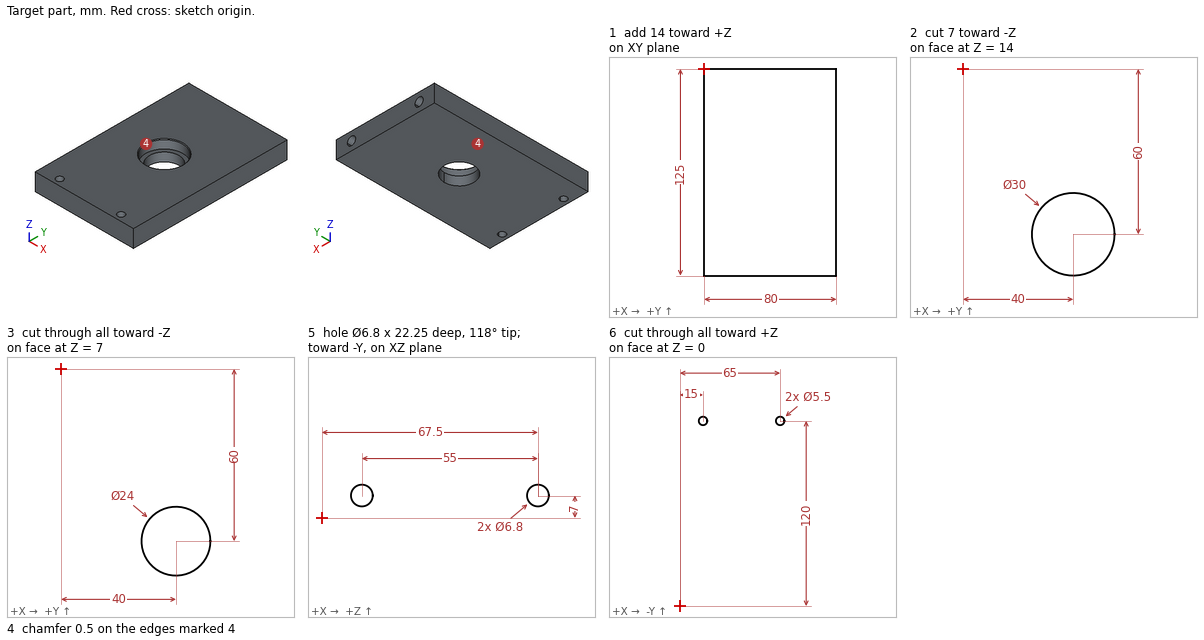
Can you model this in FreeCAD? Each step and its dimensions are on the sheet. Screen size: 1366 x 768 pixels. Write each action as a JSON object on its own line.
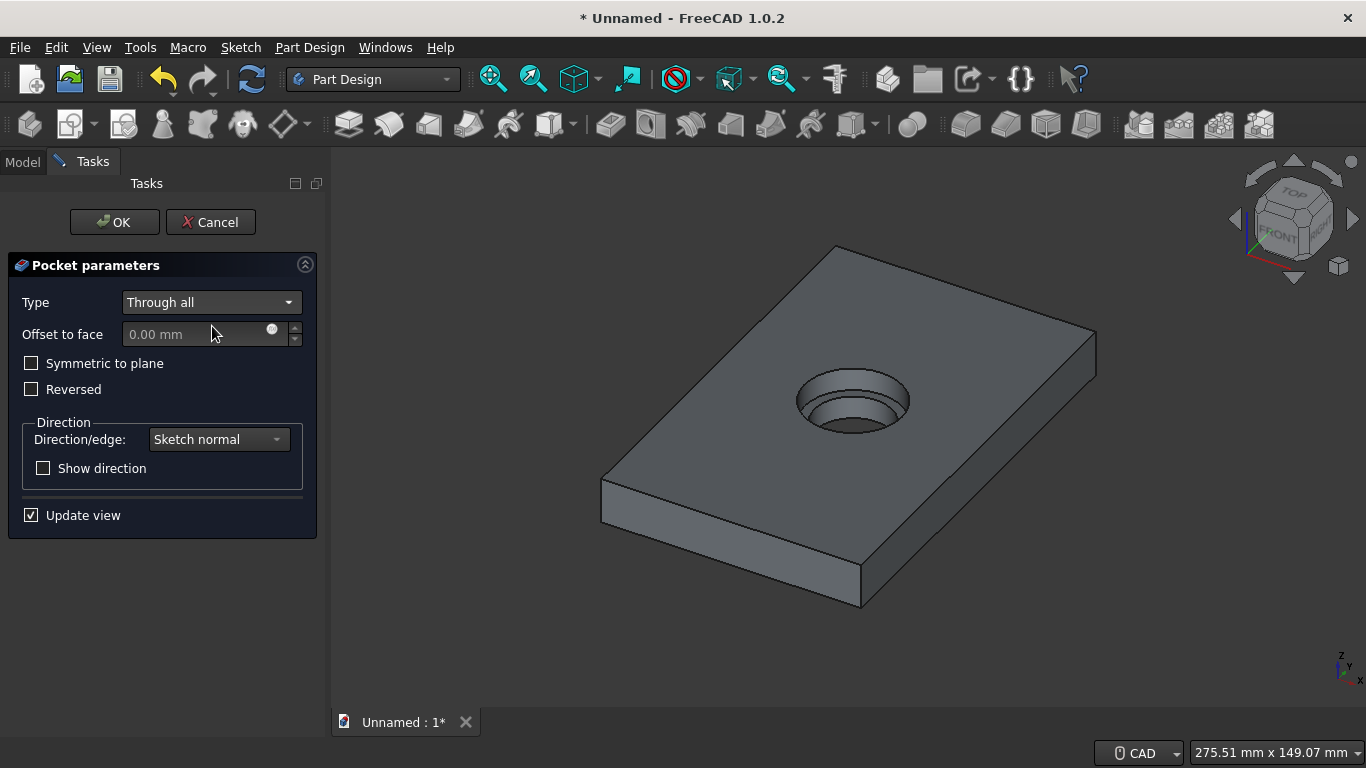
{"action": "left_click", "coordinate": [115, 222]}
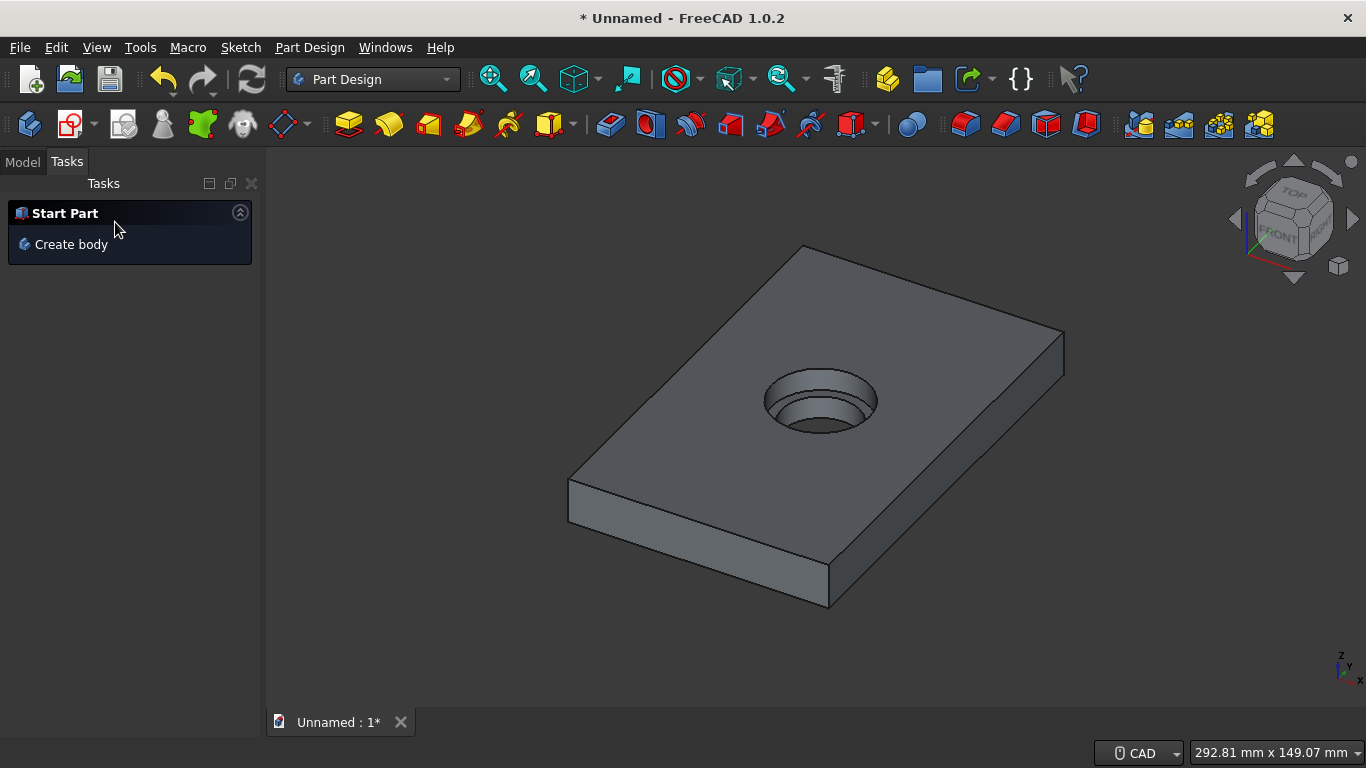
{"action": "left_click", "coordinate": [772, 384]}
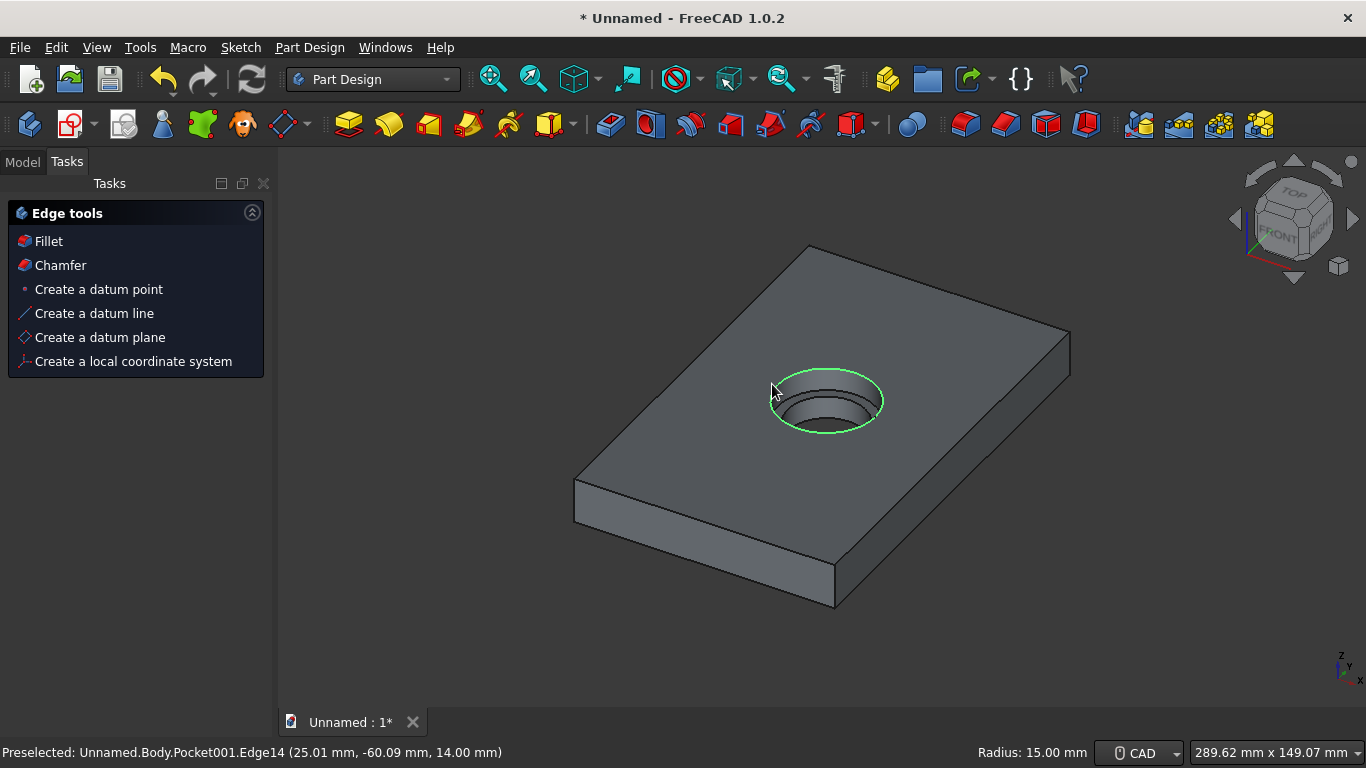
{"action": "left_click", "coordinate": [1006, 124]}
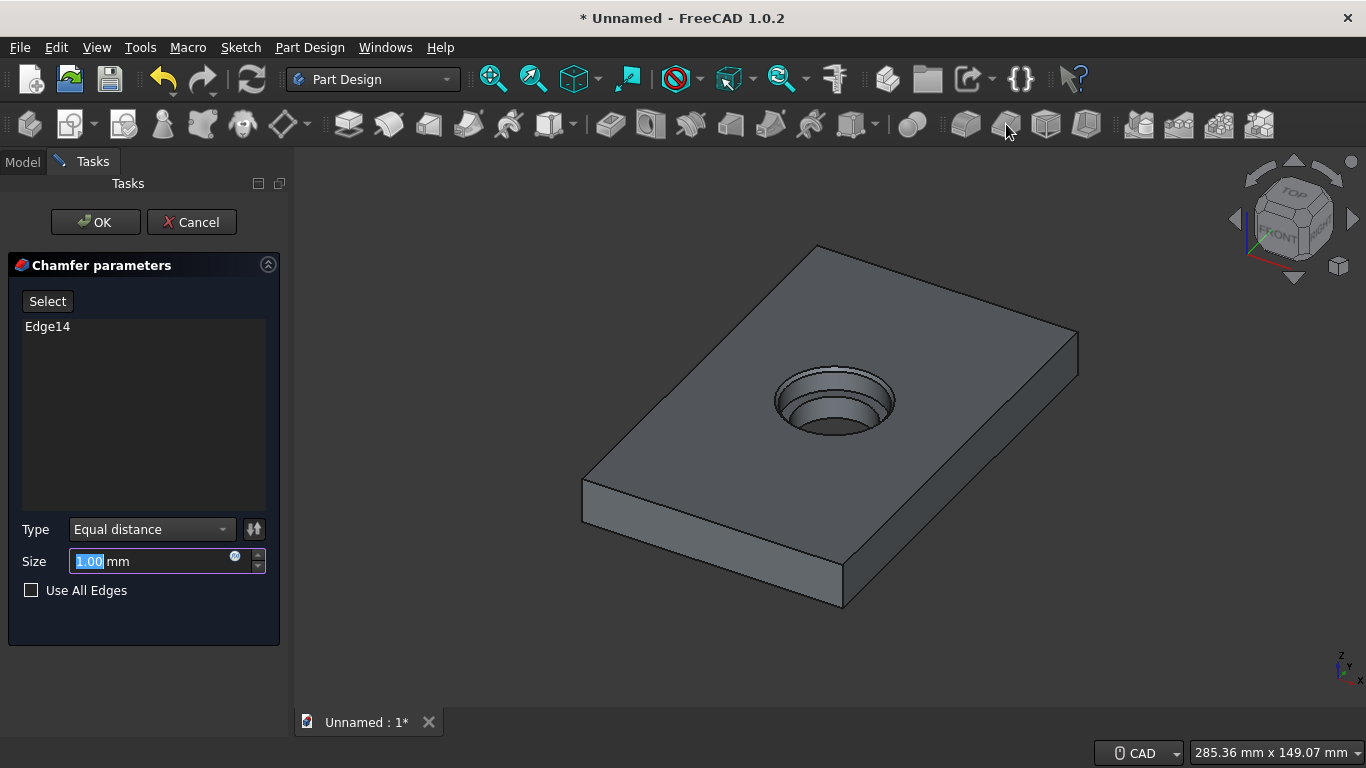
{"action": "type", "text": "0.5"}
{"action": "key", "text": "Tab"}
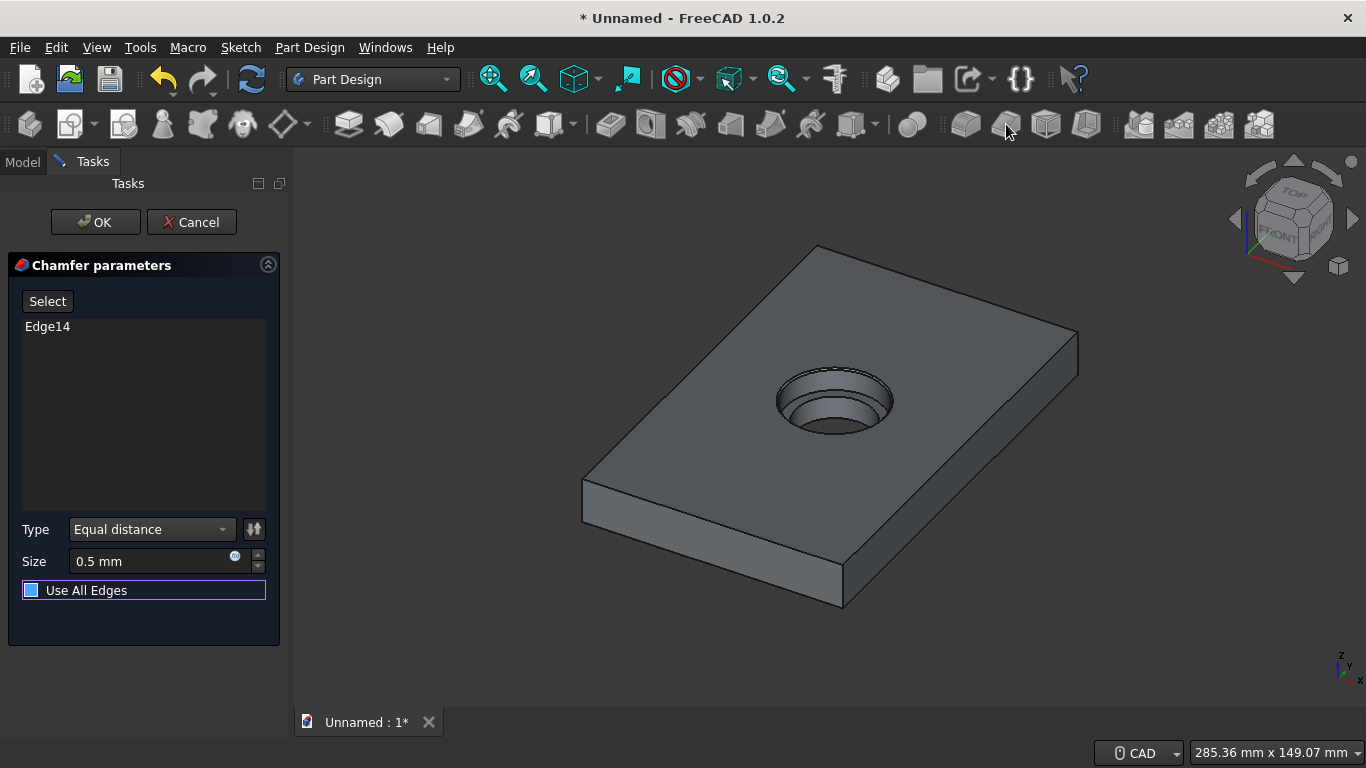
{"action": "left_click", "coordinate": [96, 222]}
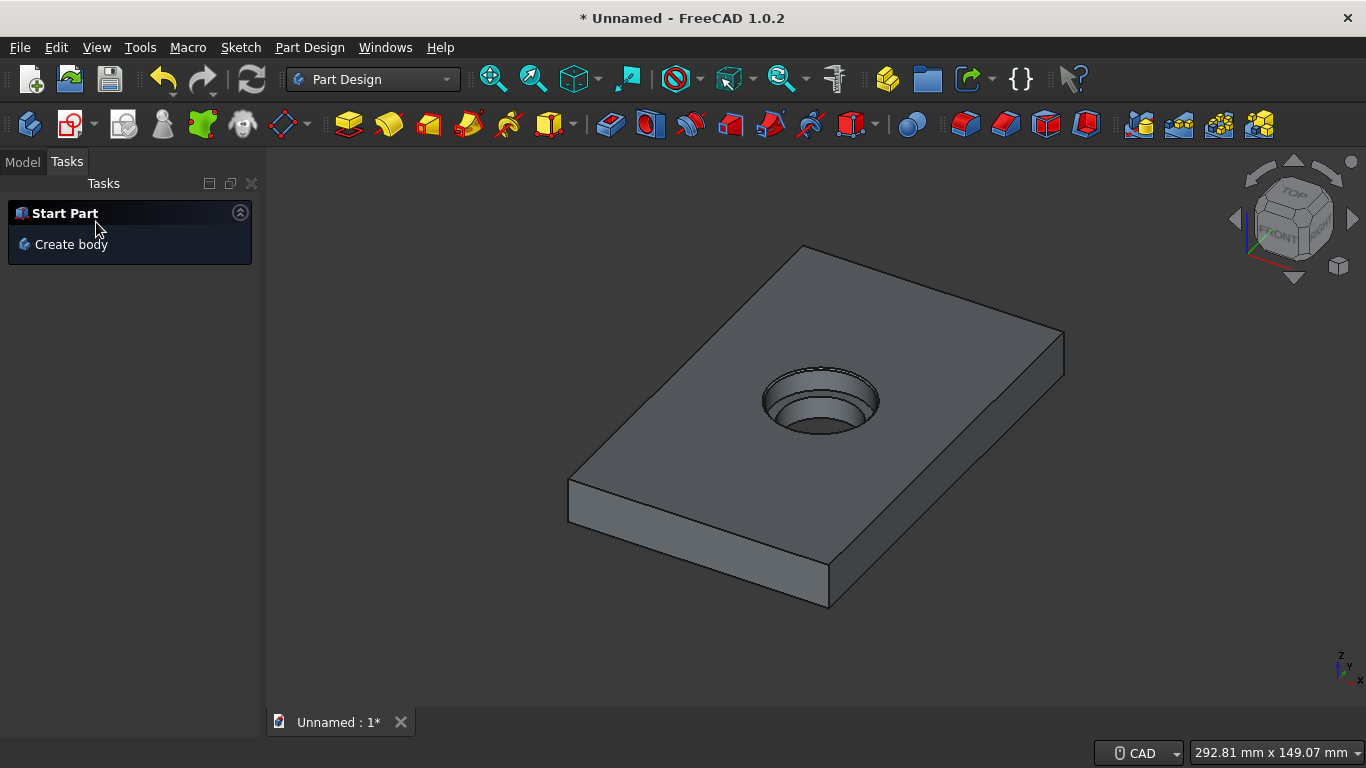
{"action": "left_click", "coordinate": [70, 124]}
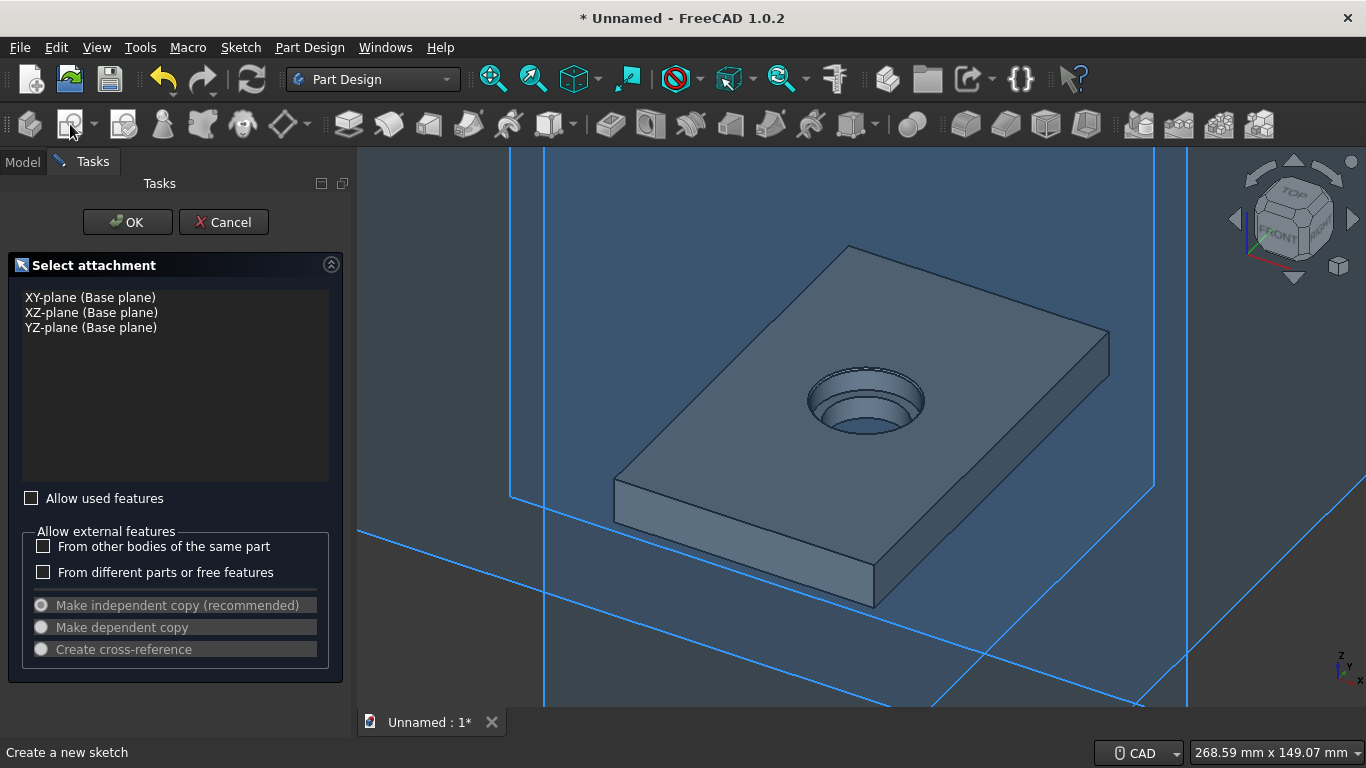
{"action": "left_click", "coordinate": [82, 312]}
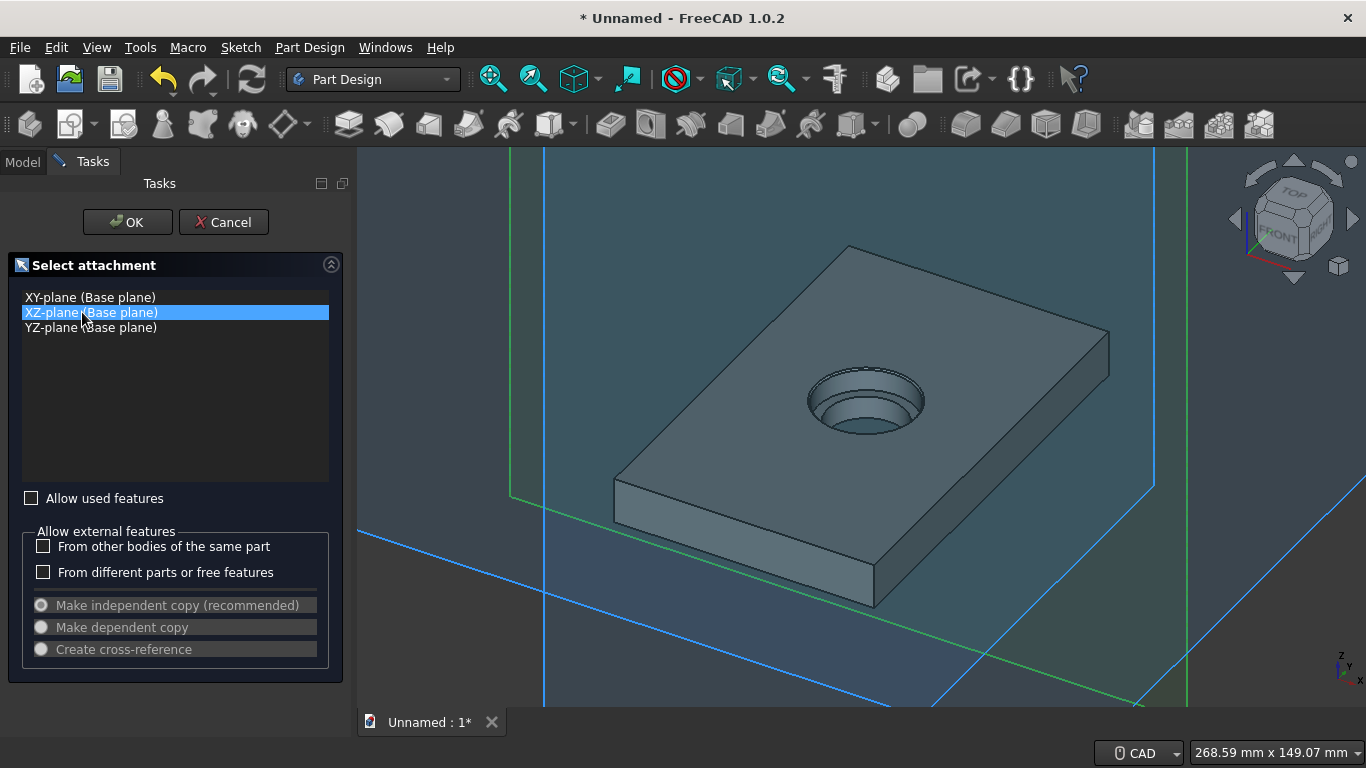
{"action": "left_click", "coordinate": [128, 222]}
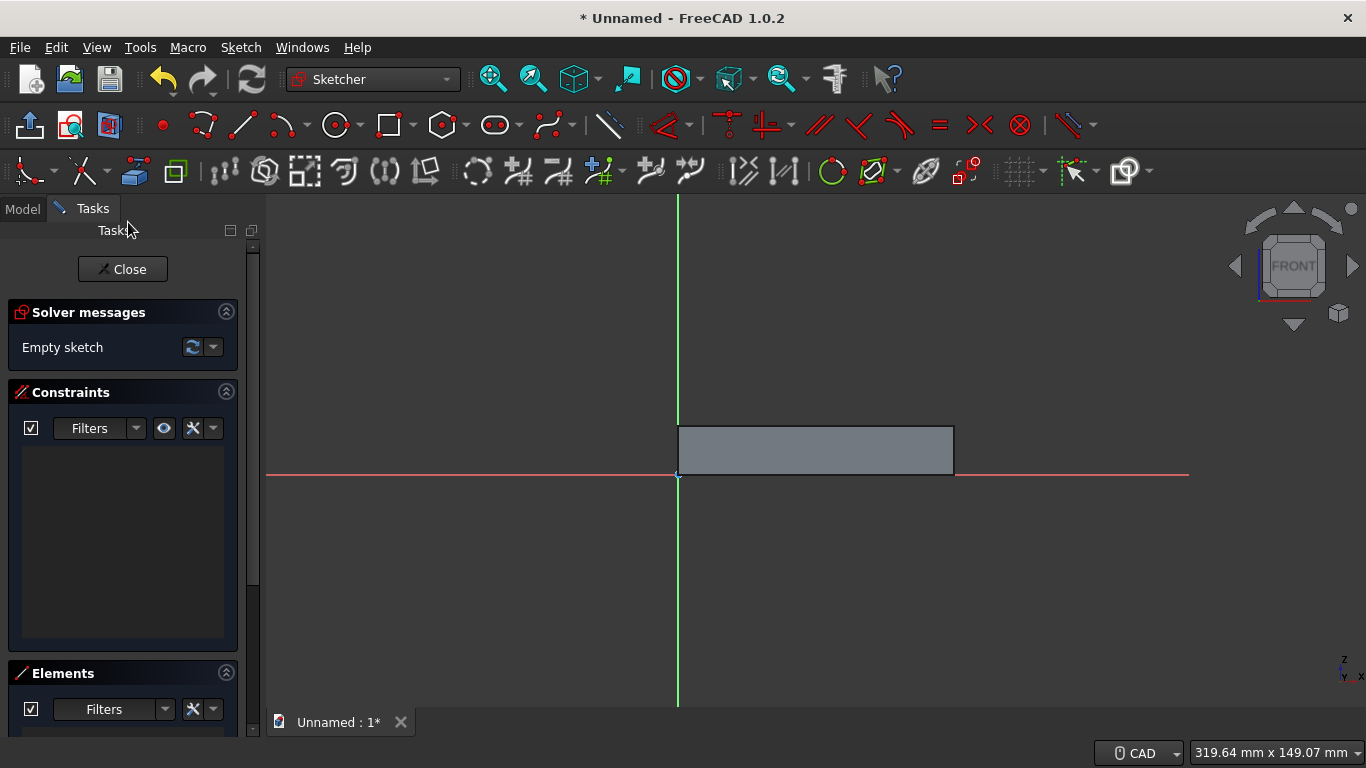
{"action": "left_click", "coordinate": [110, 126]}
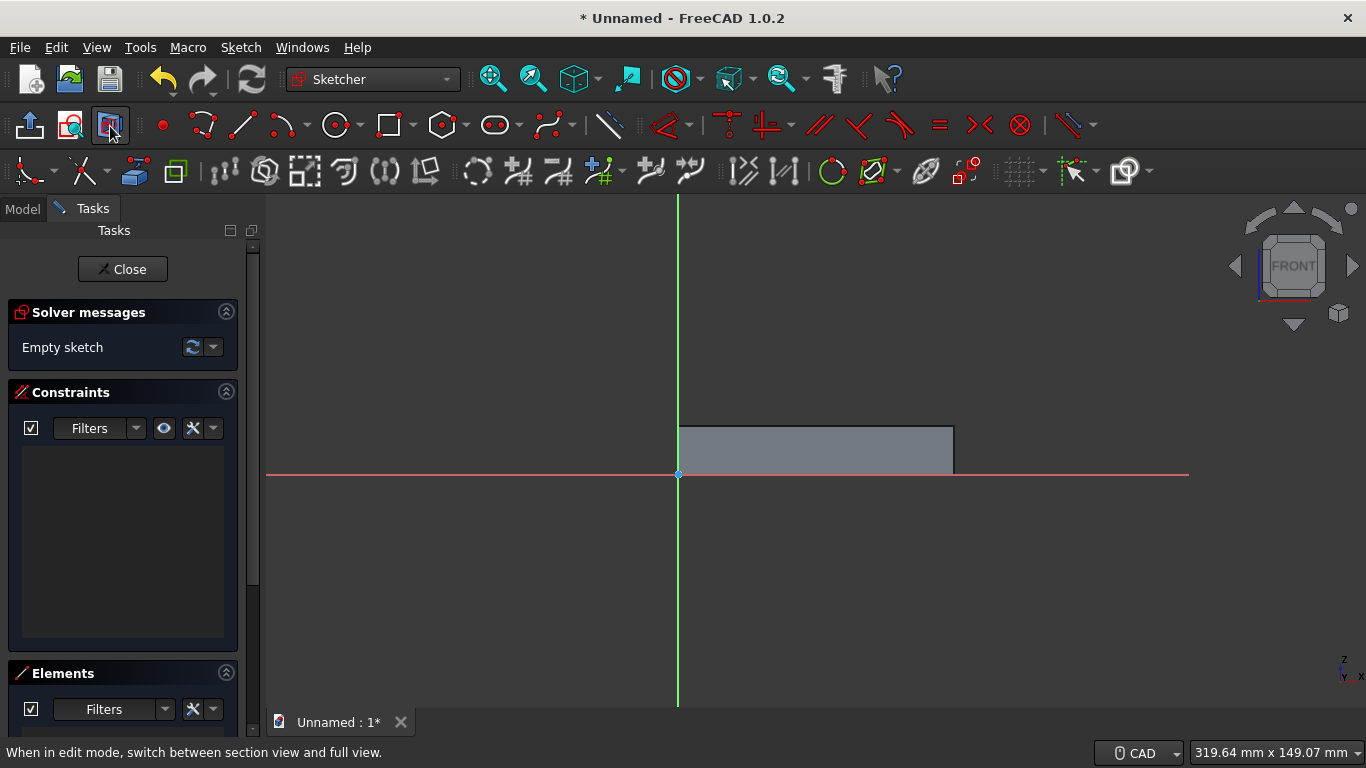
{"action": "scroll", "coordinate": [831, 460], "scroll_direction": "up", "scroll_amount": 5}